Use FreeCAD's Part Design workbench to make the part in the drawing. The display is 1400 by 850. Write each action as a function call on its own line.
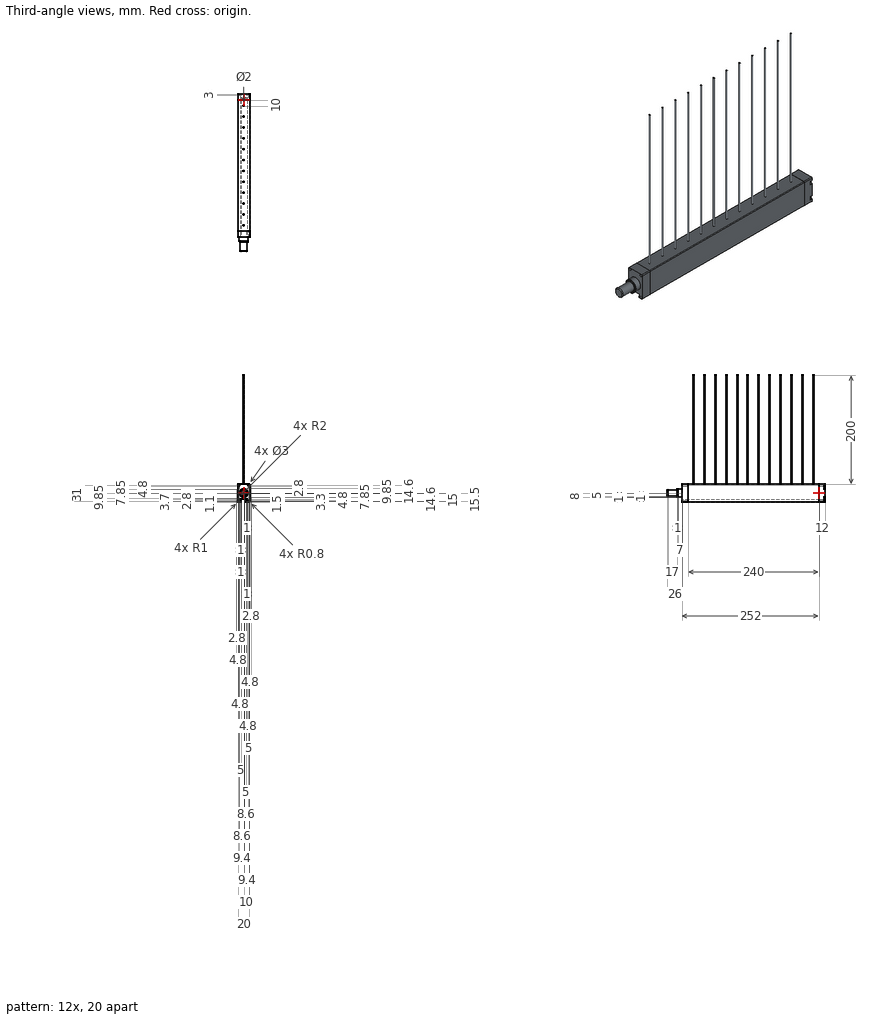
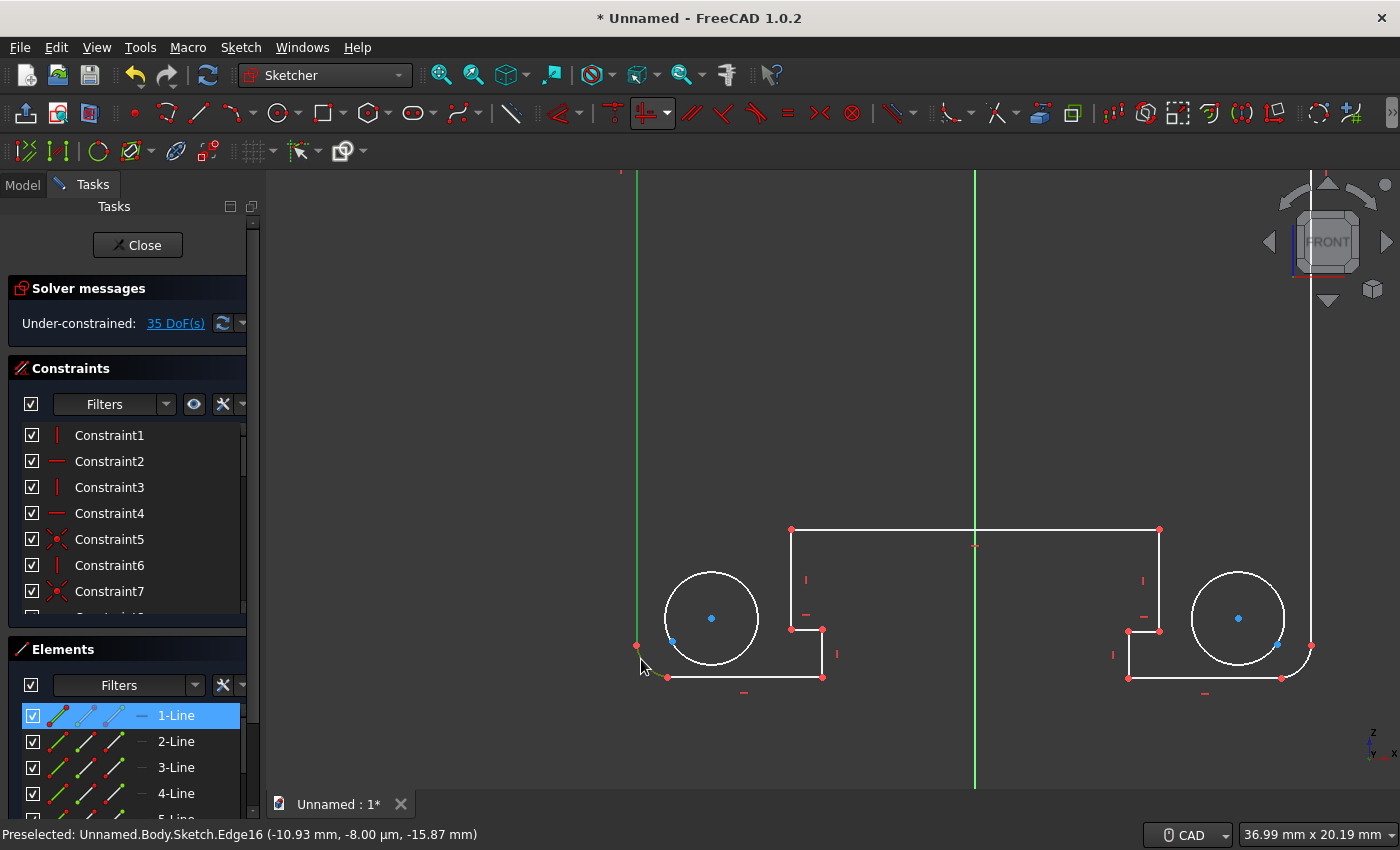
click(756, 114)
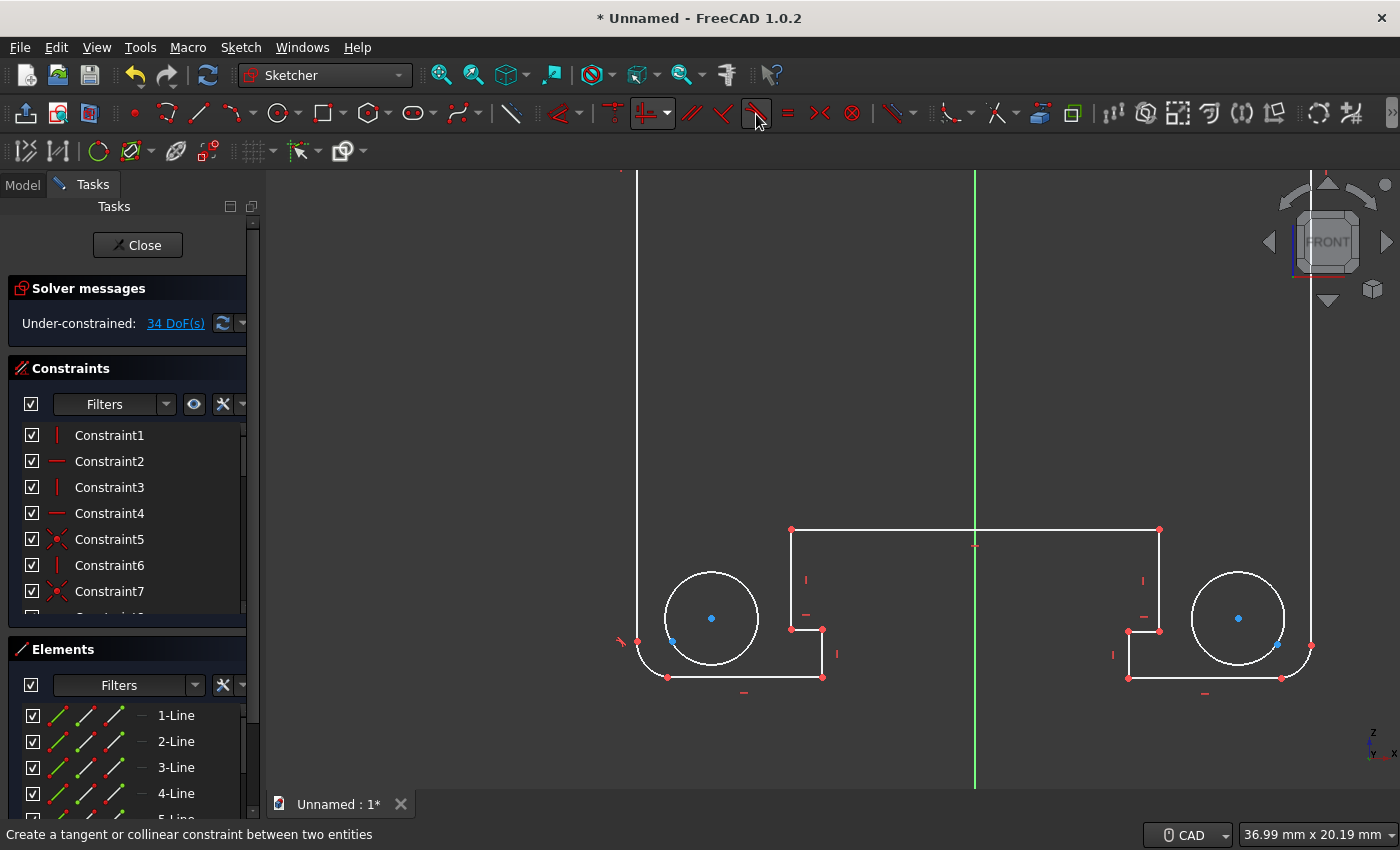
scroll(642, 660, down, 5)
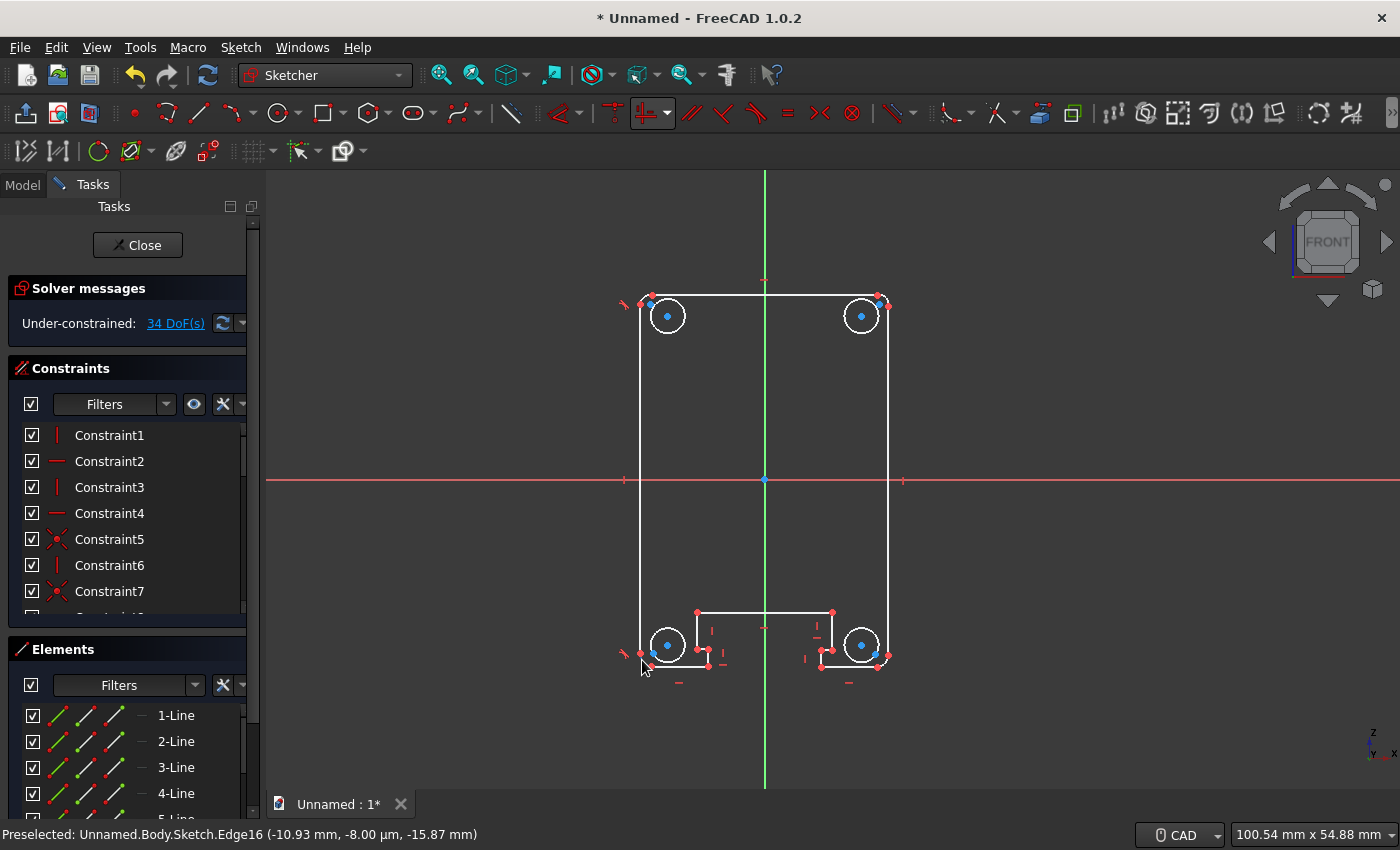
click(720, 295)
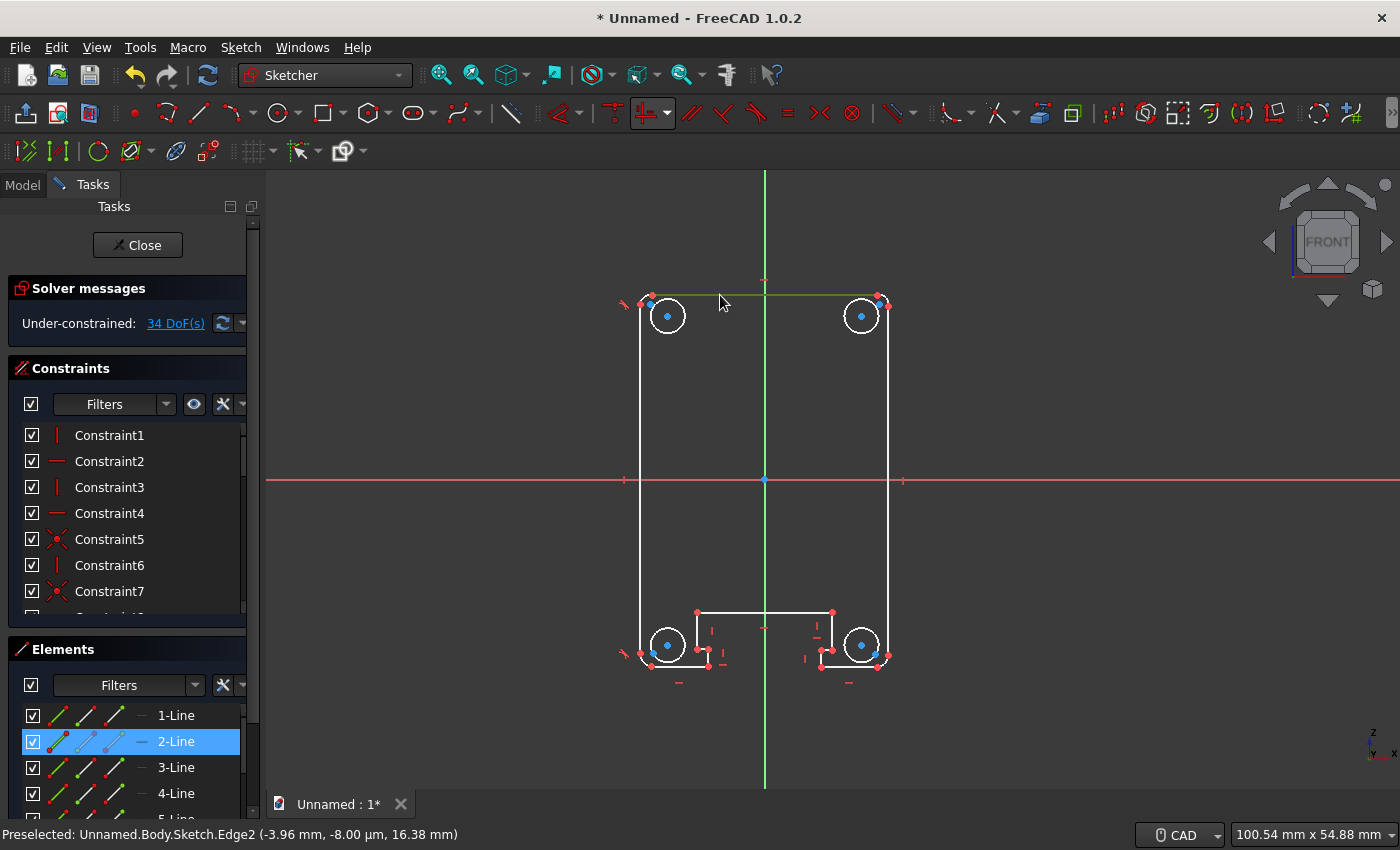
scroll(644, 297, up, 3)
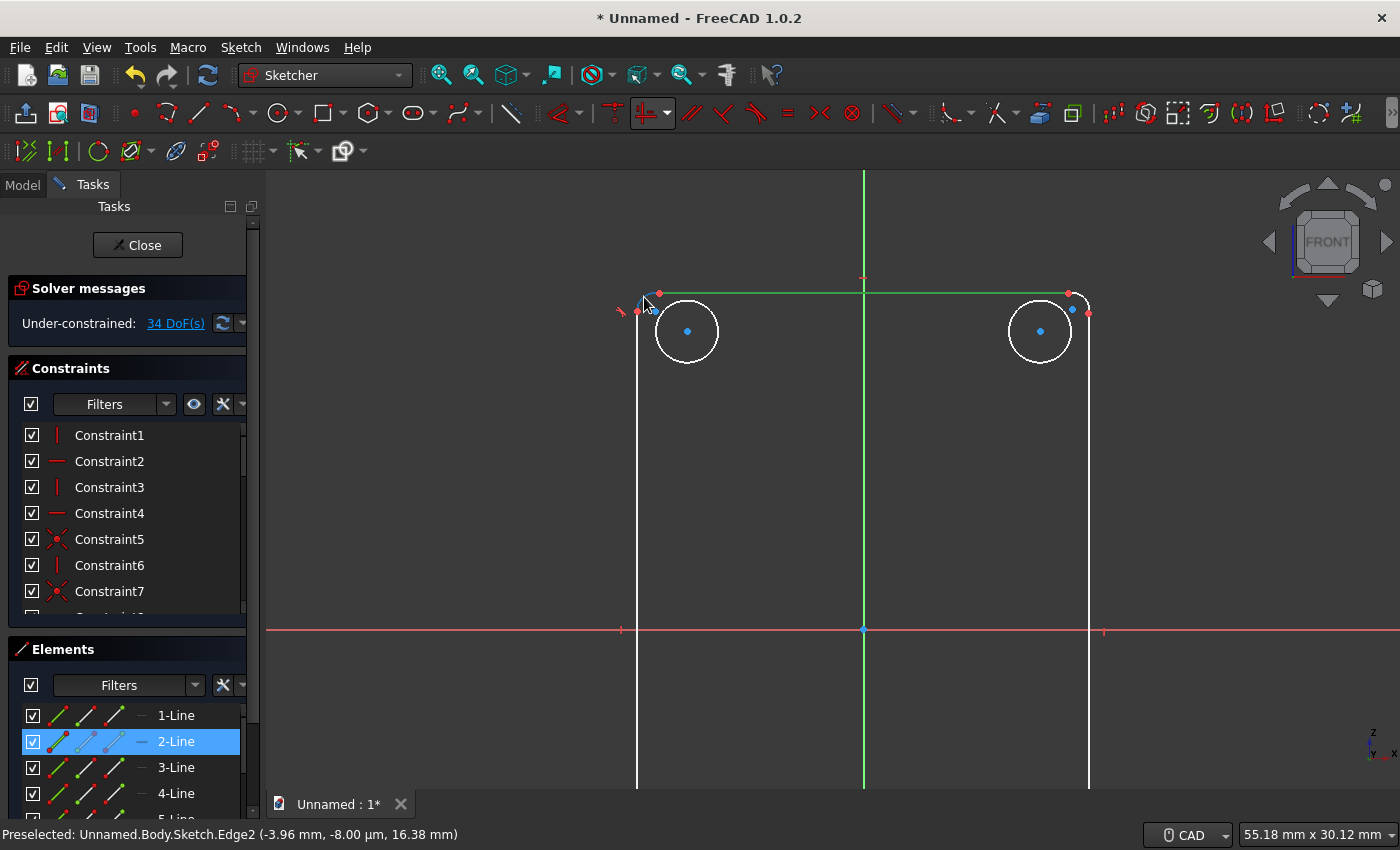
click(644, 297)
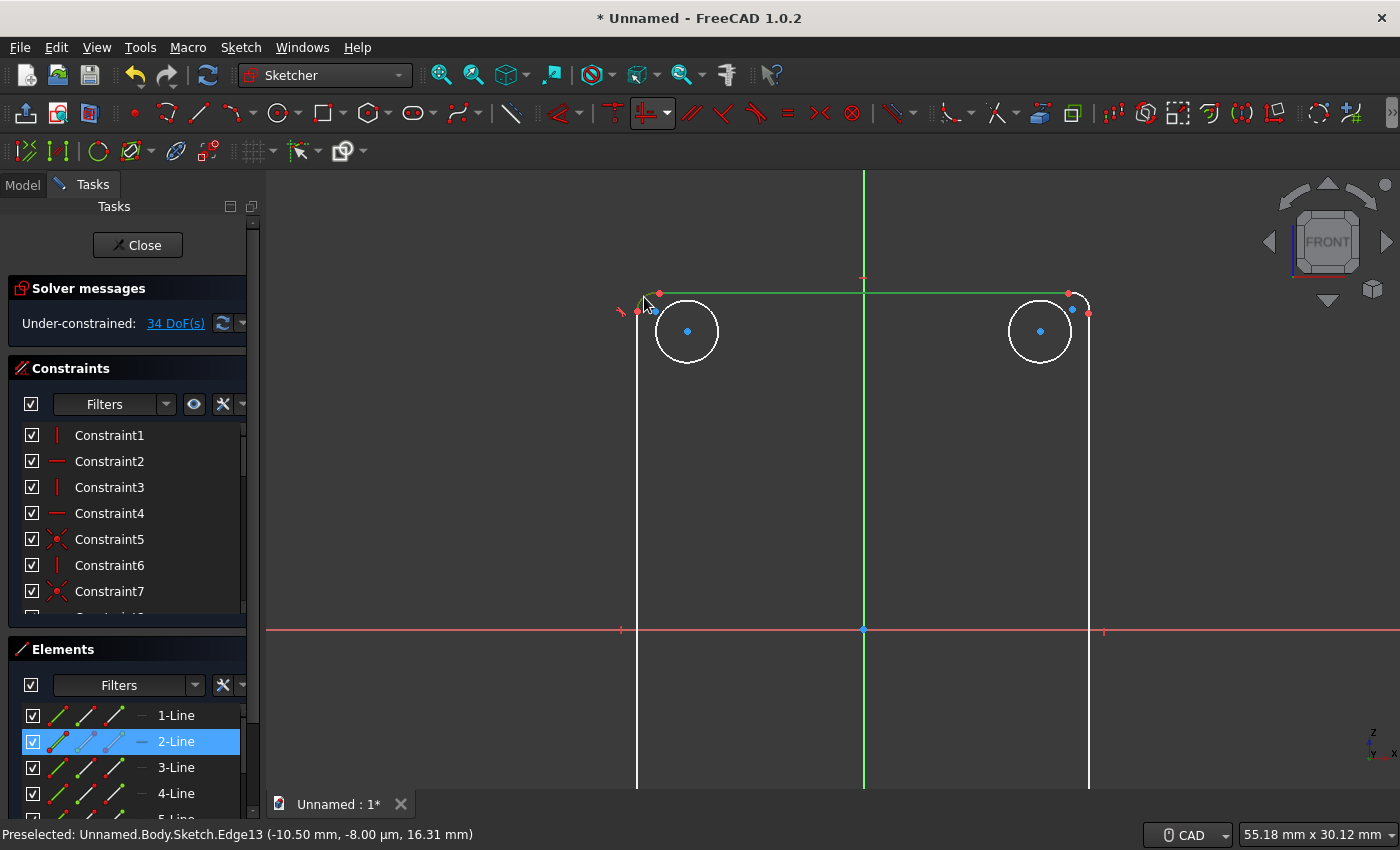
key(t)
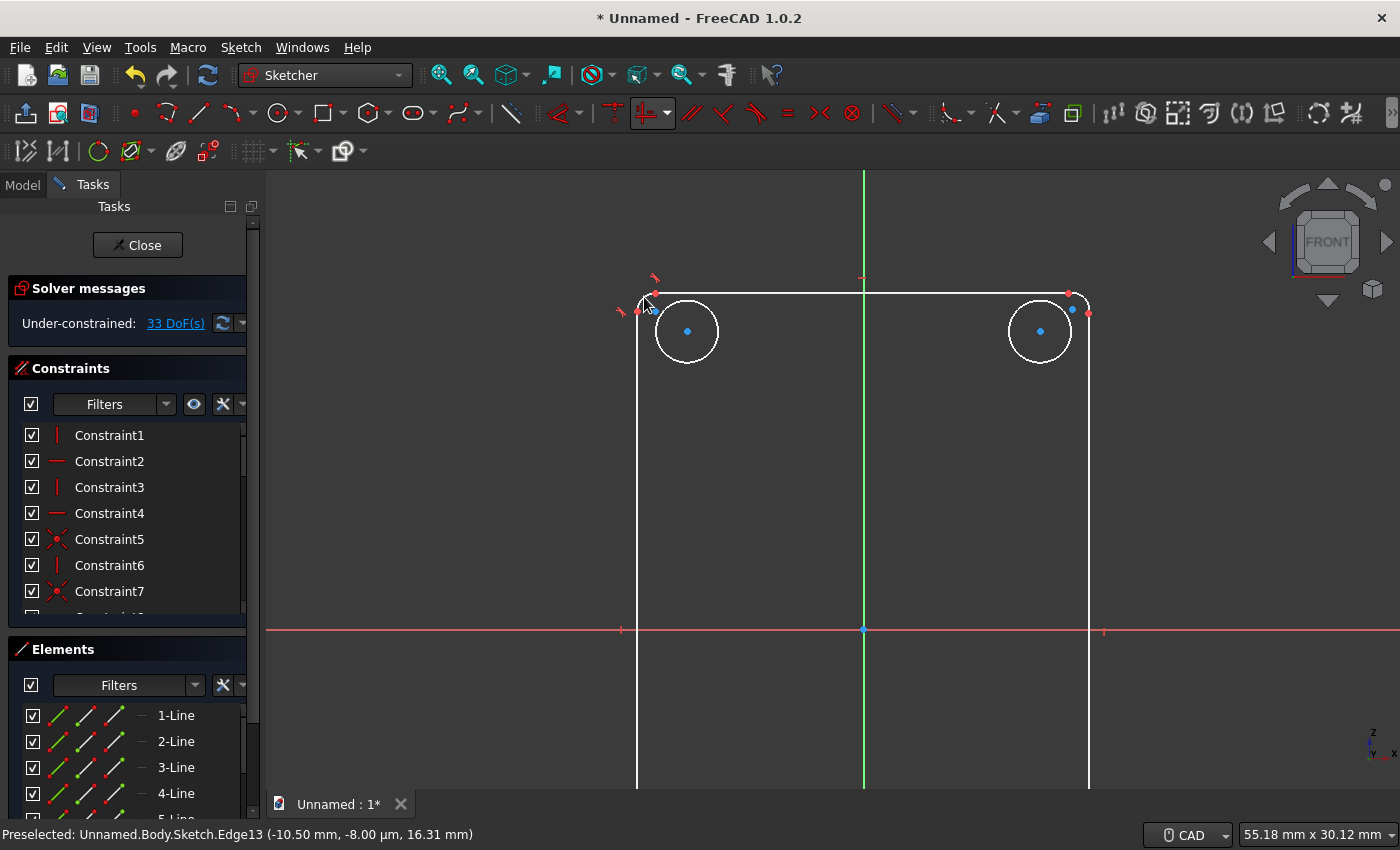
click(780, 293)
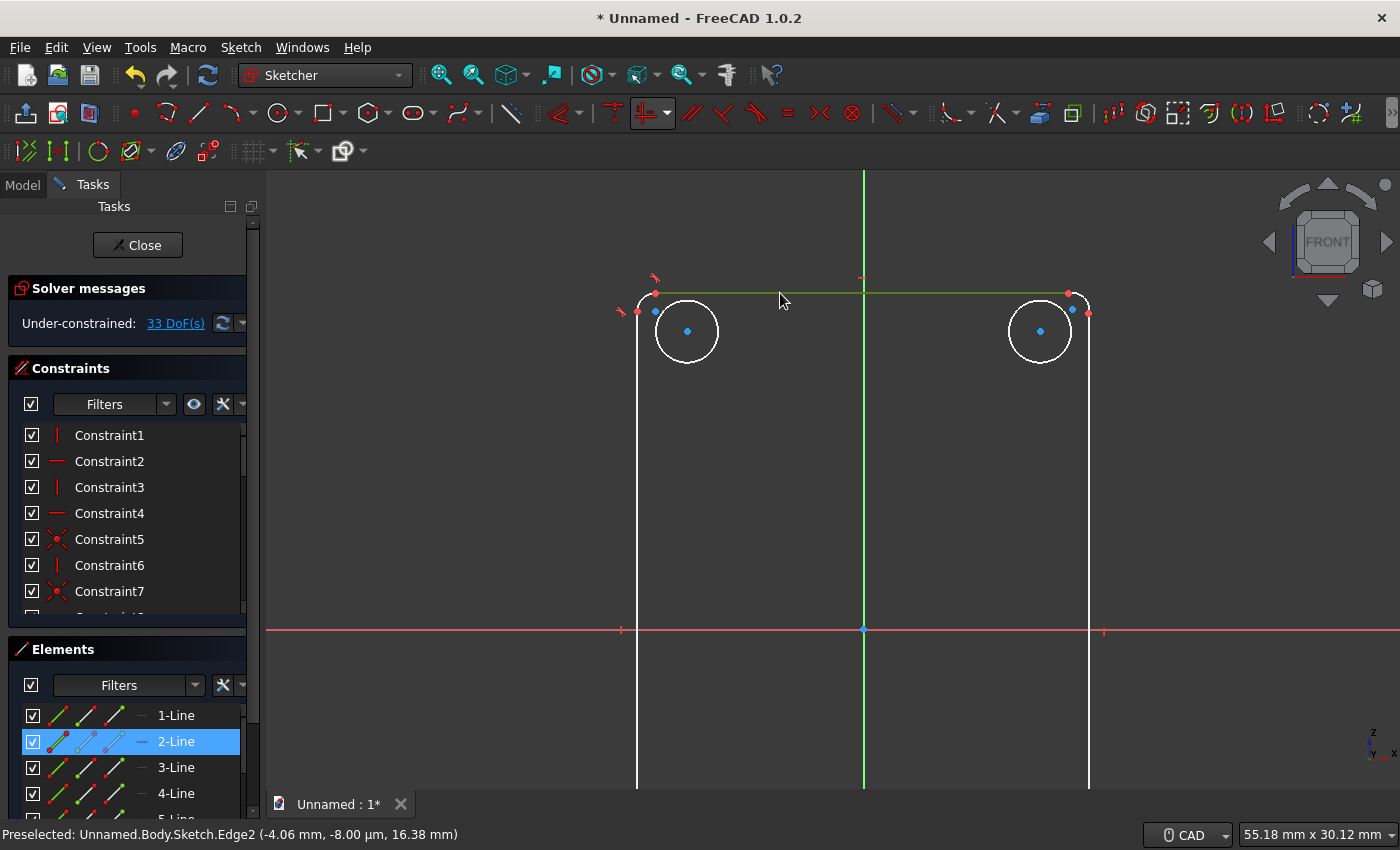
scroll(1088, 303, up, 2)